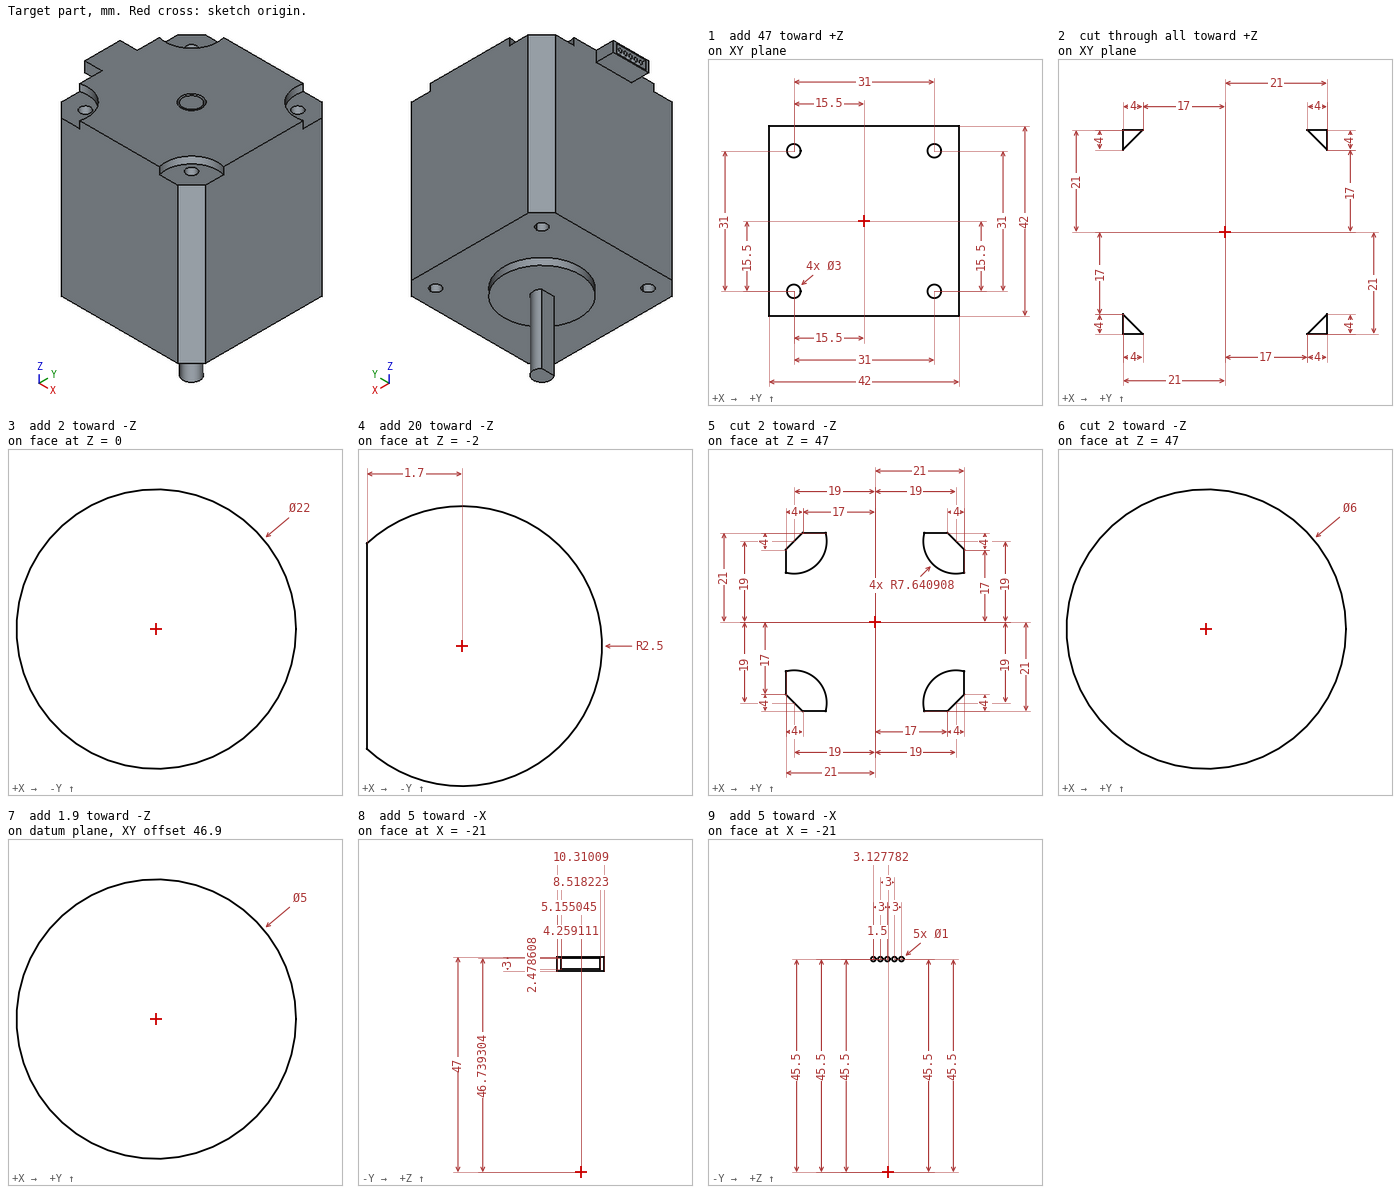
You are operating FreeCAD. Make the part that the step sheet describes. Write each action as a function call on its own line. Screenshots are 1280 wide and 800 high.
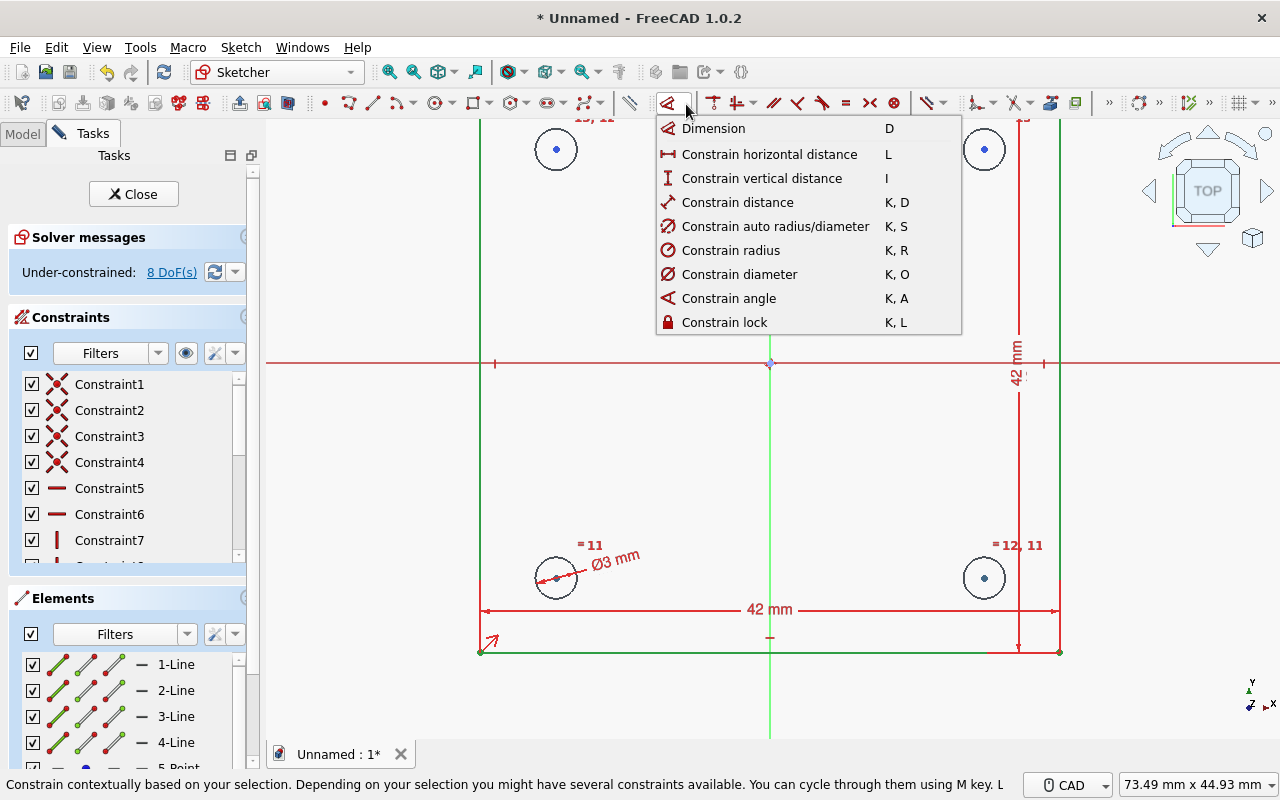
click(809, 154)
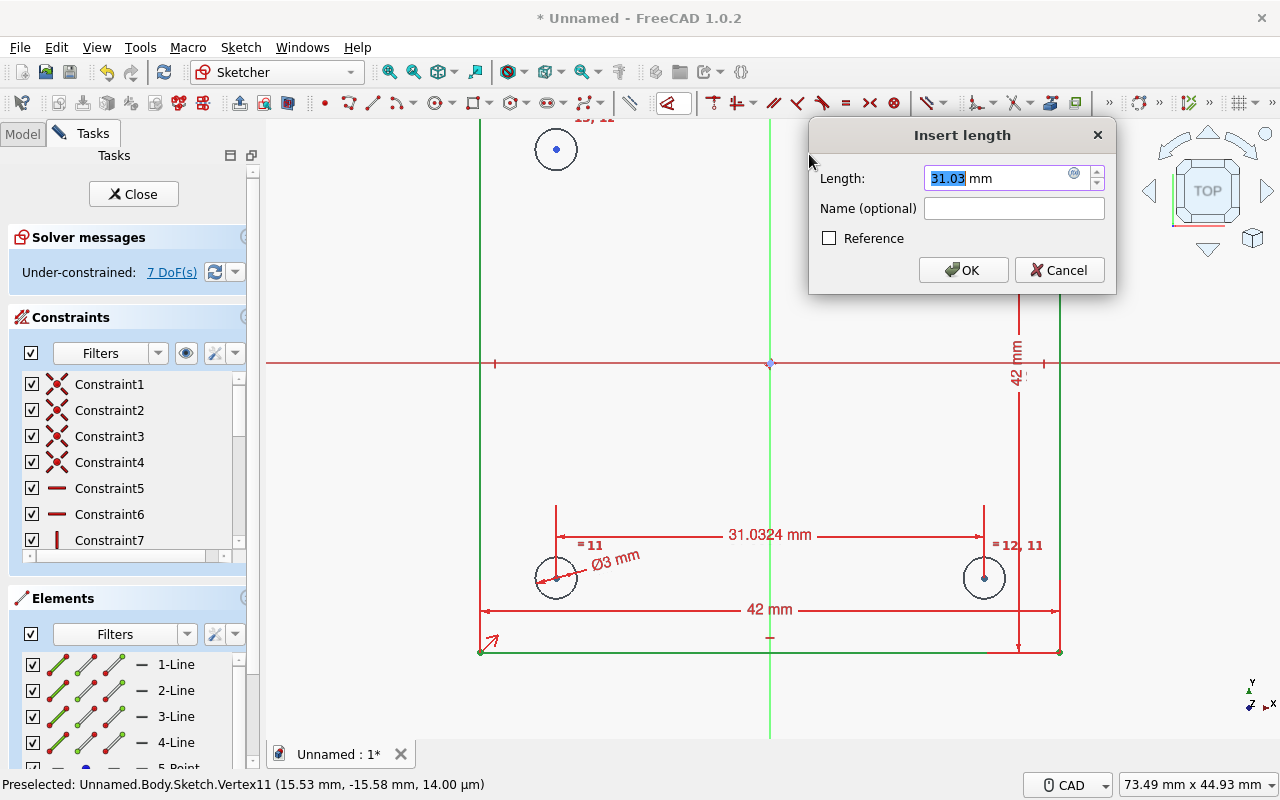
text(31)
key(Return)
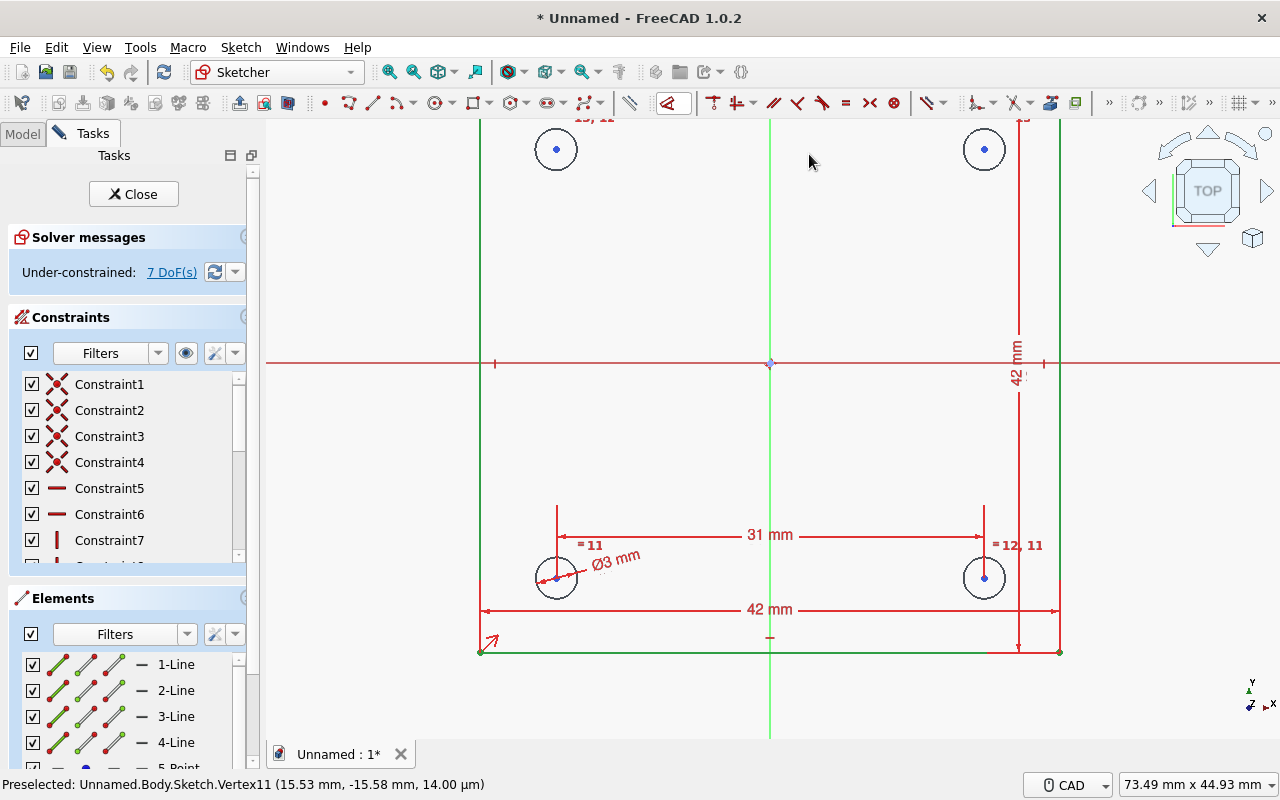
click(557, 578)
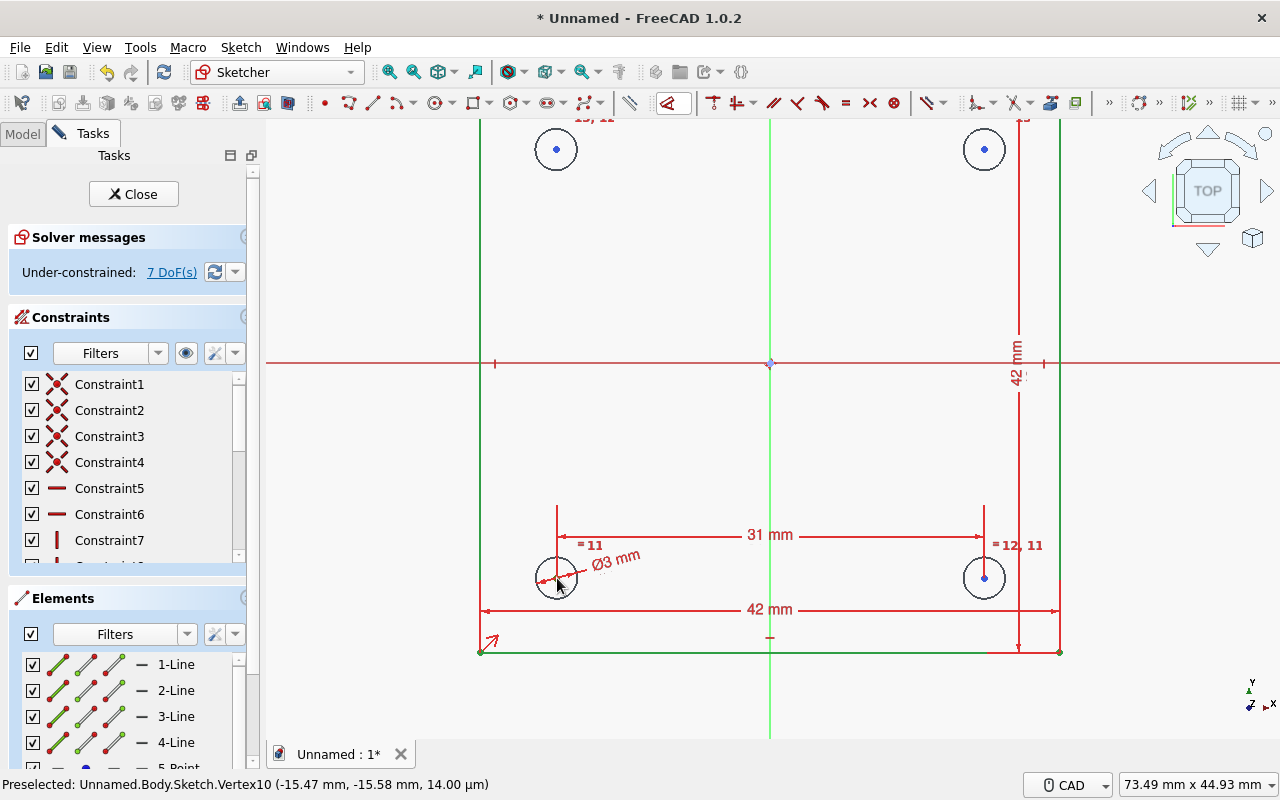
click(556, 150)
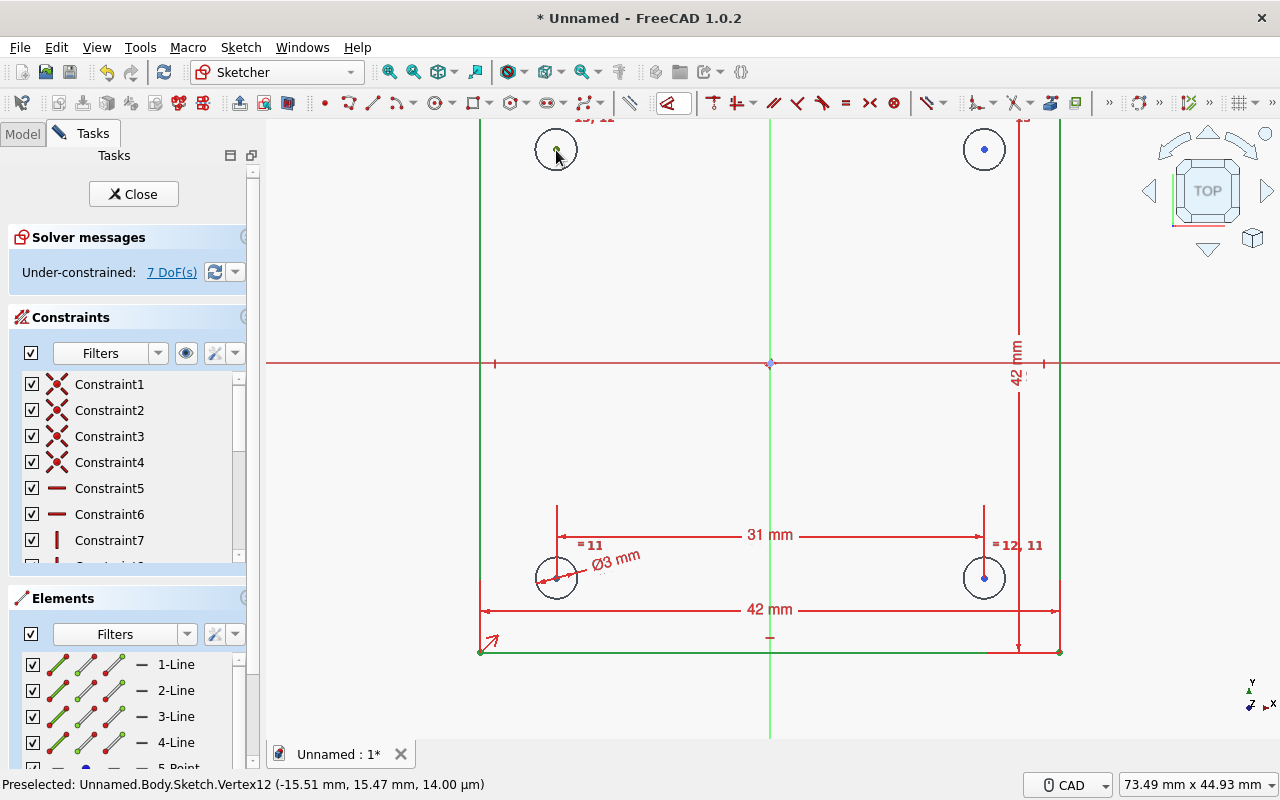
click(686, 104)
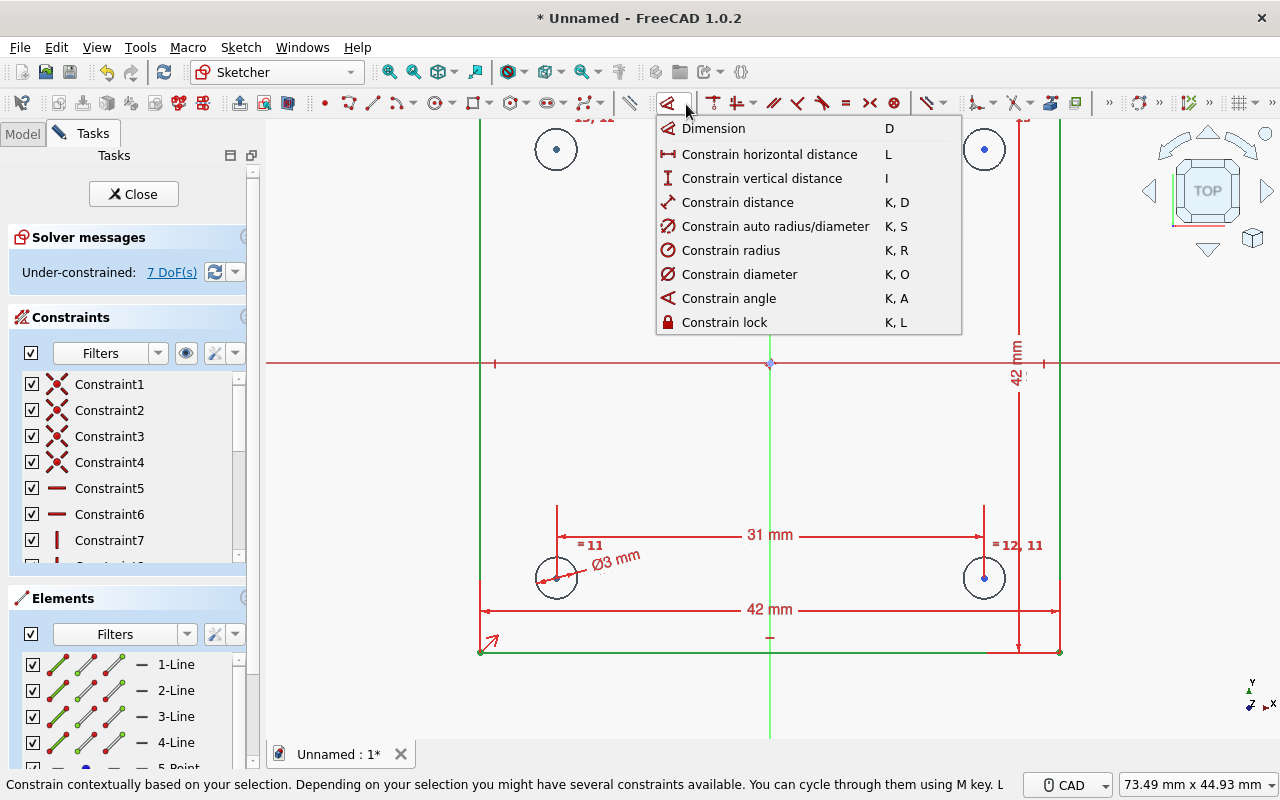
click(809, 178)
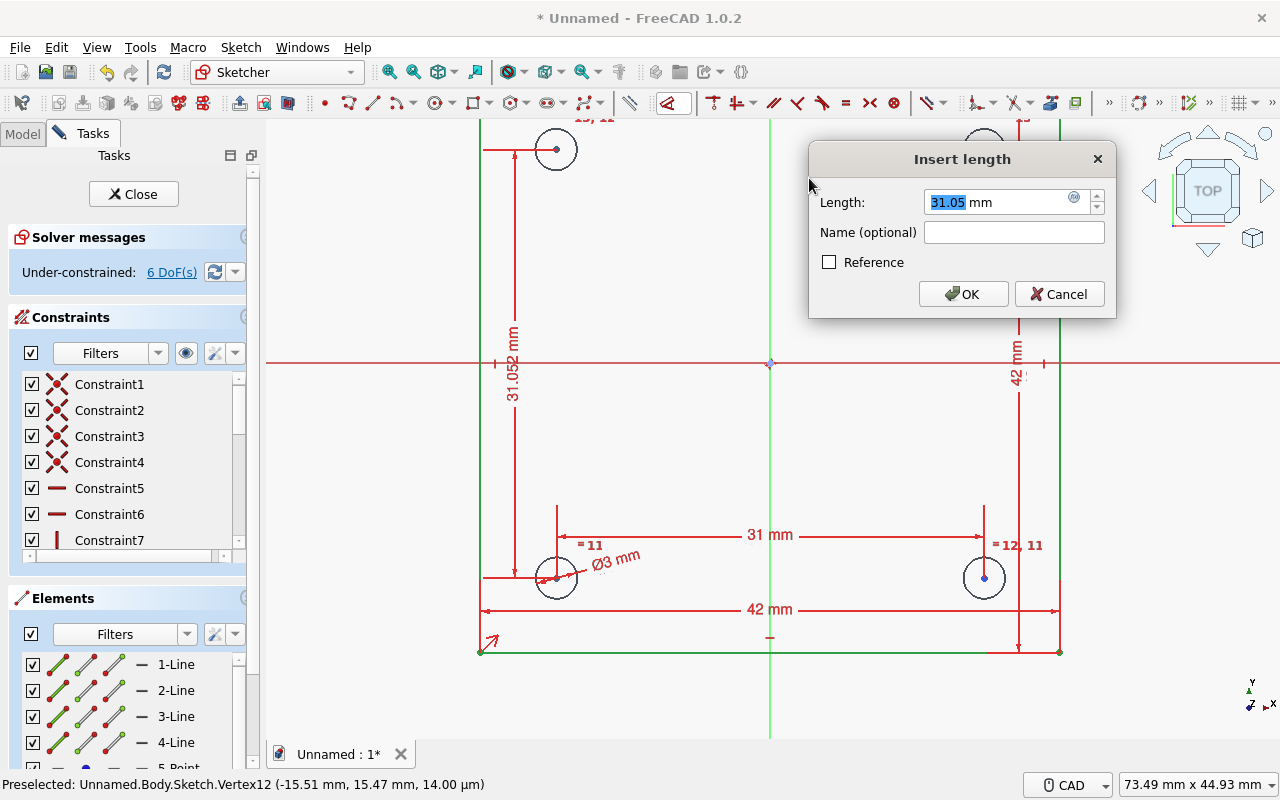
text(31)
key(Return)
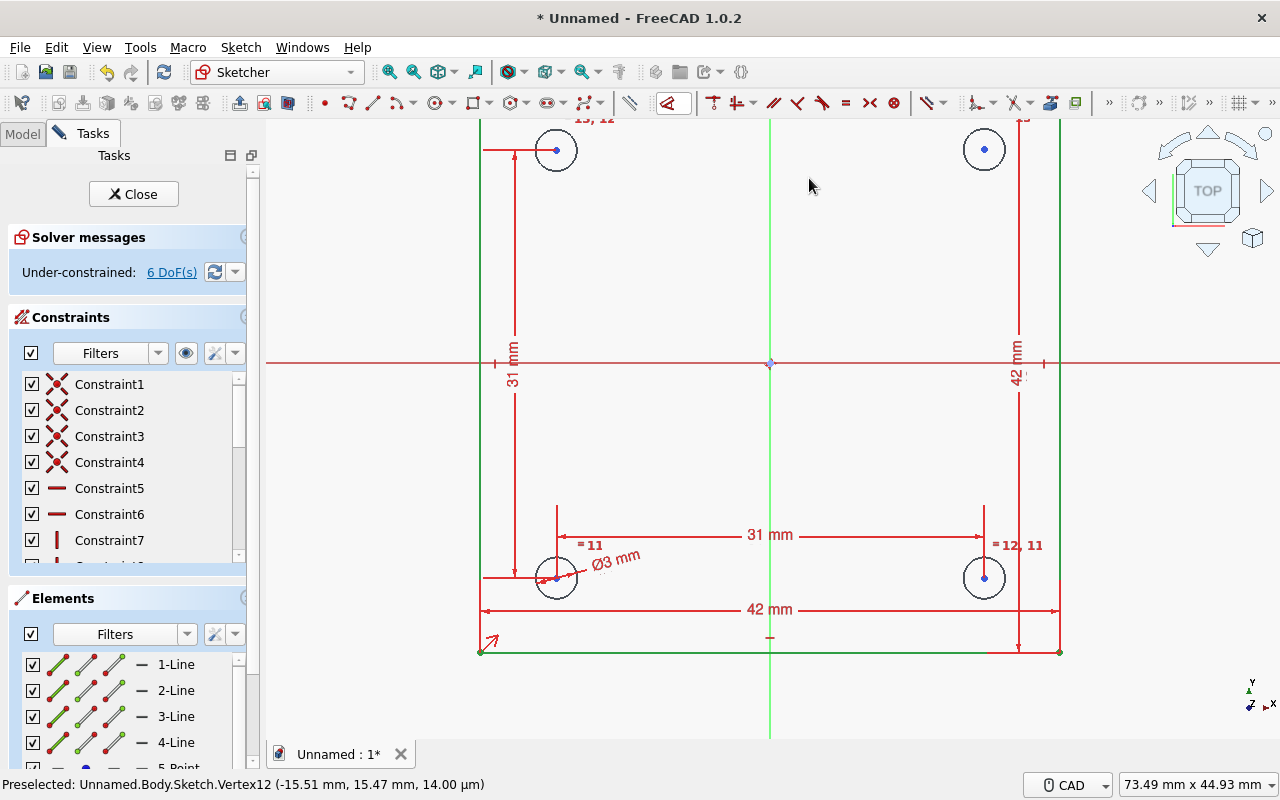
click(556, 150)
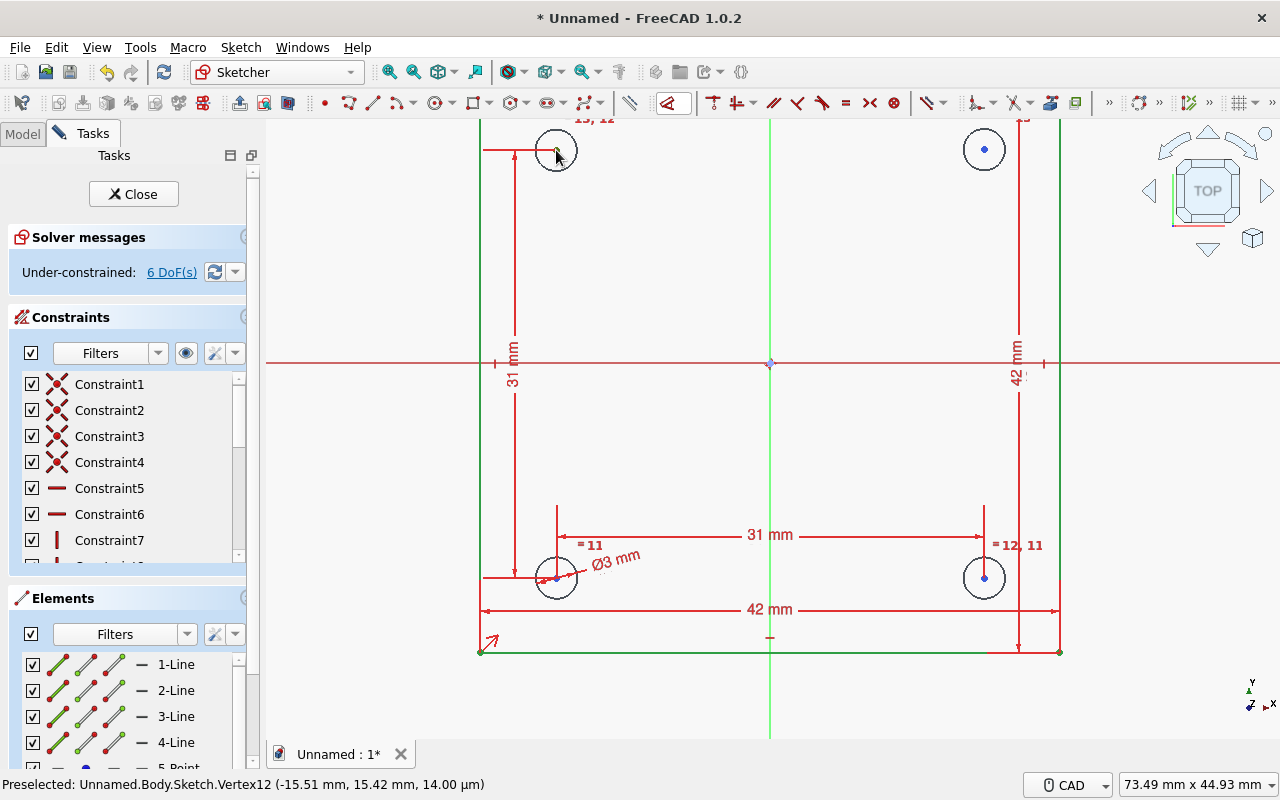
click(984, 150)